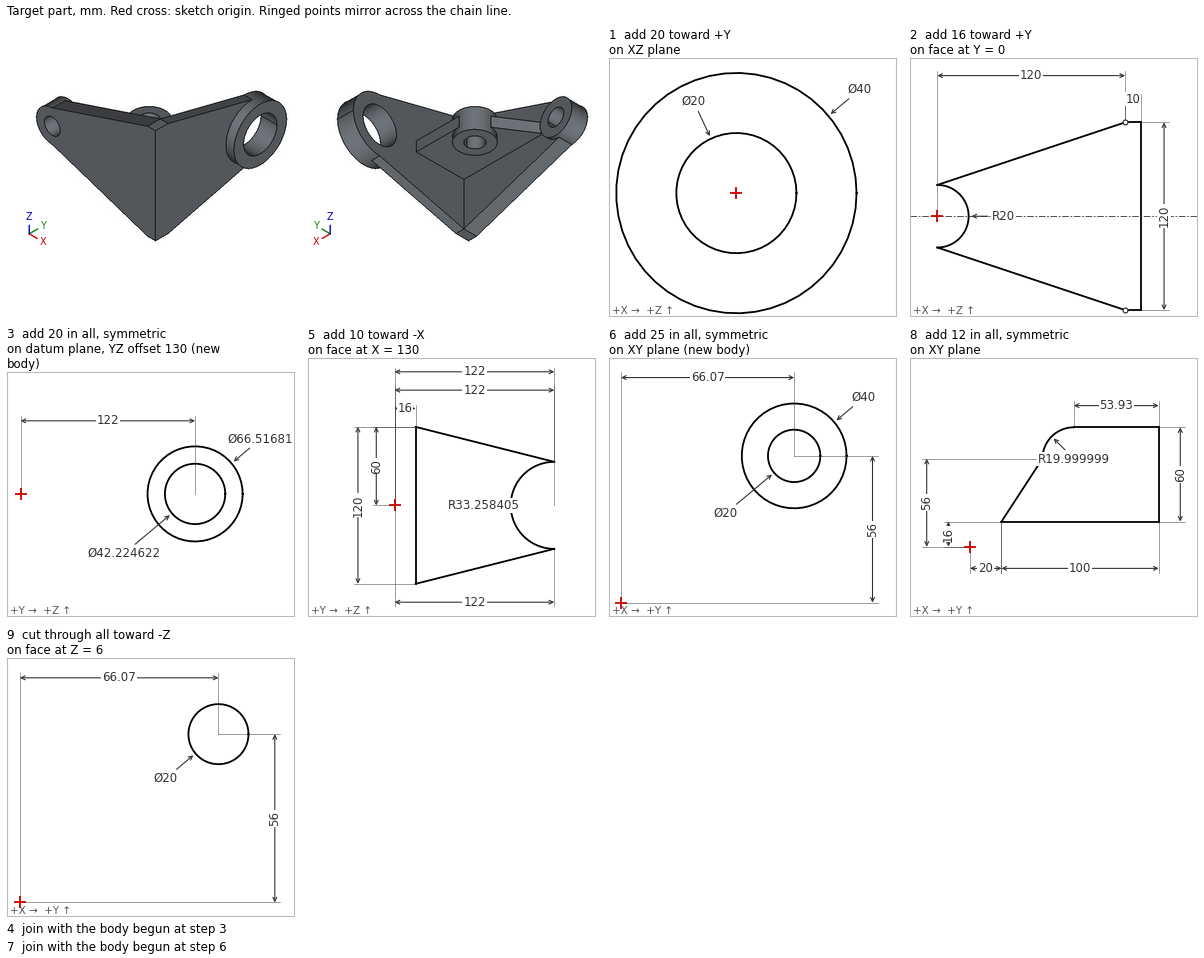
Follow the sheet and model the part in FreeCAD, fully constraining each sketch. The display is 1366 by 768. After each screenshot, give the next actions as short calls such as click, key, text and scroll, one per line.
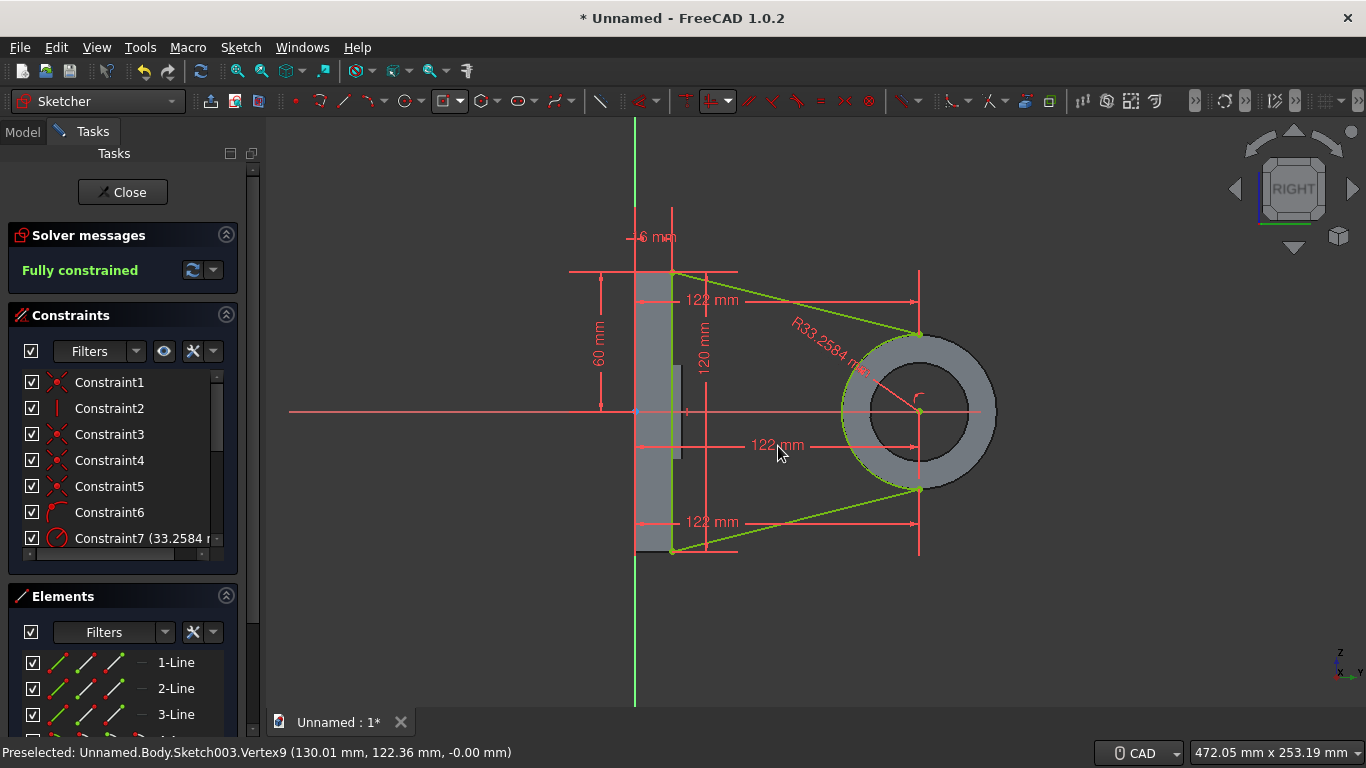
click(123, 192)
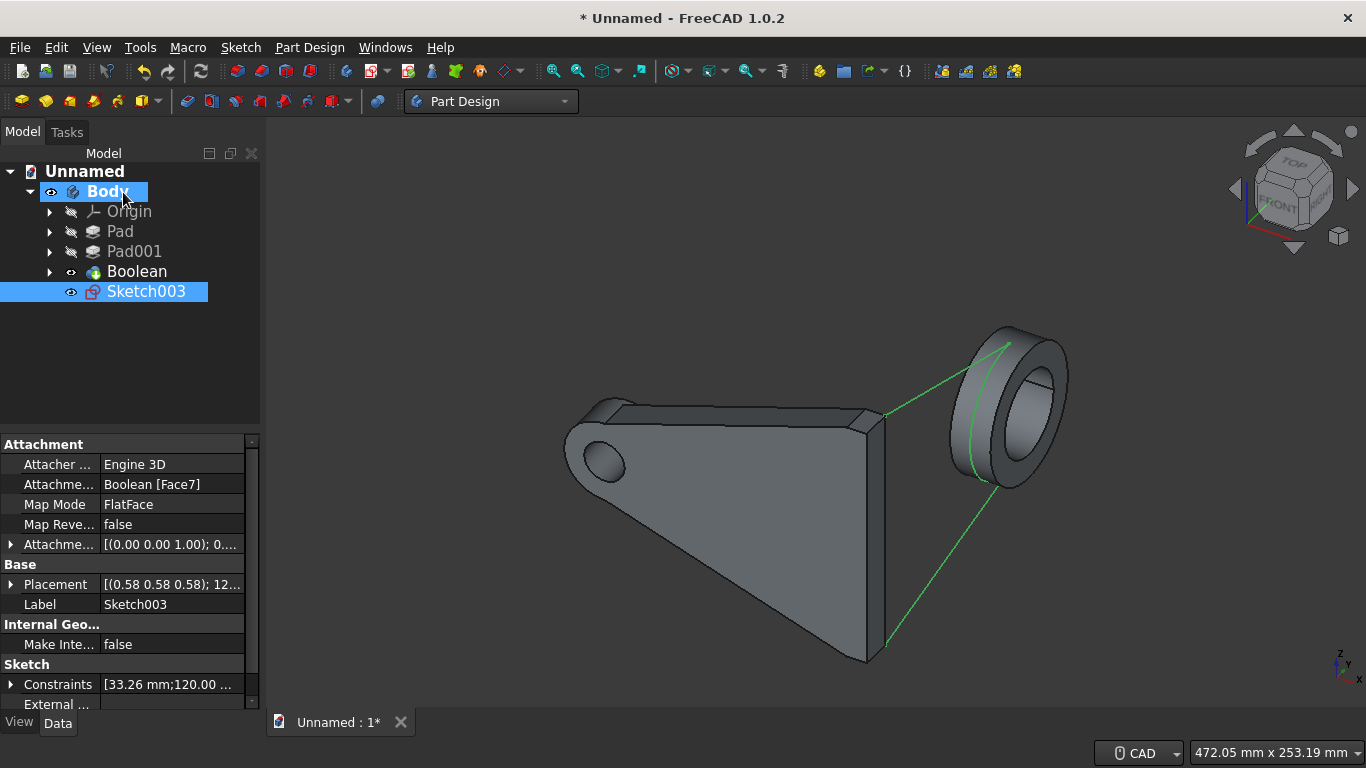
click(22, 102)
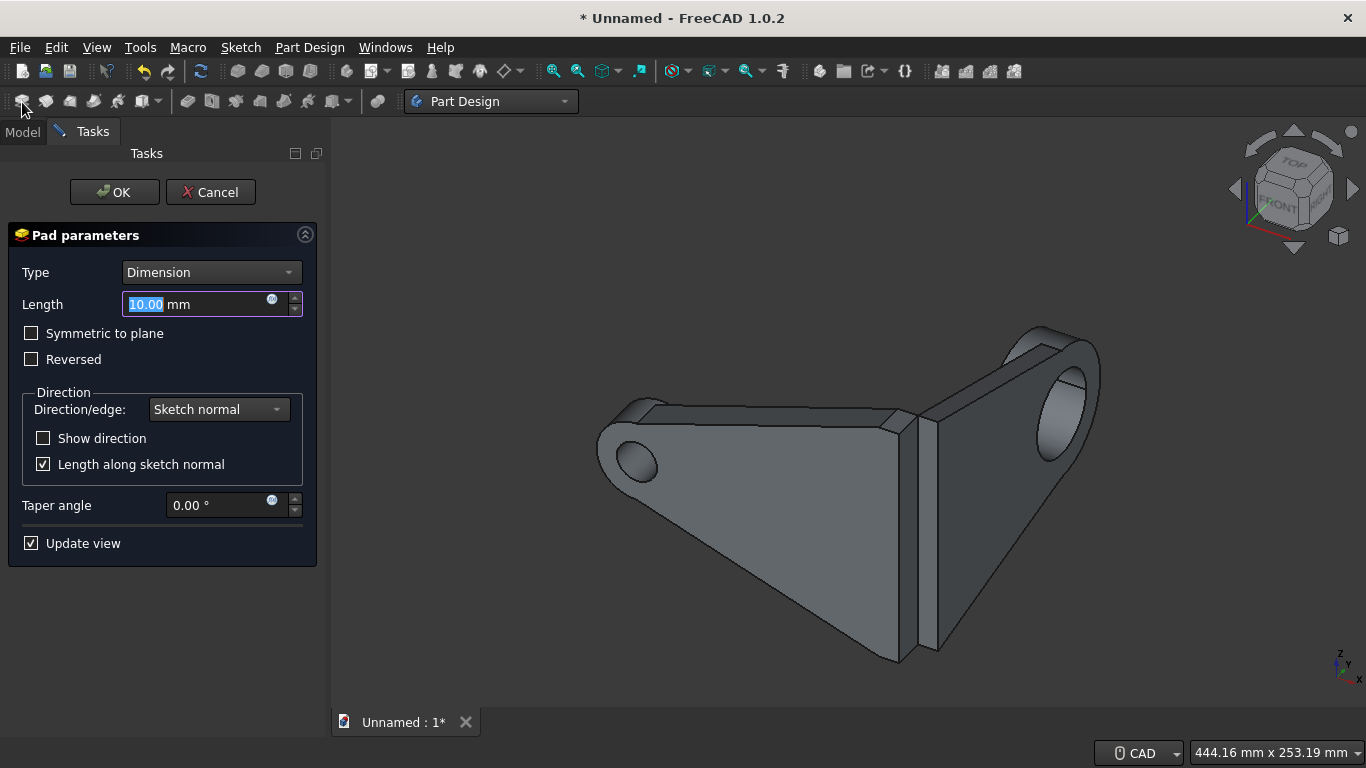
text(10)
key(Tab)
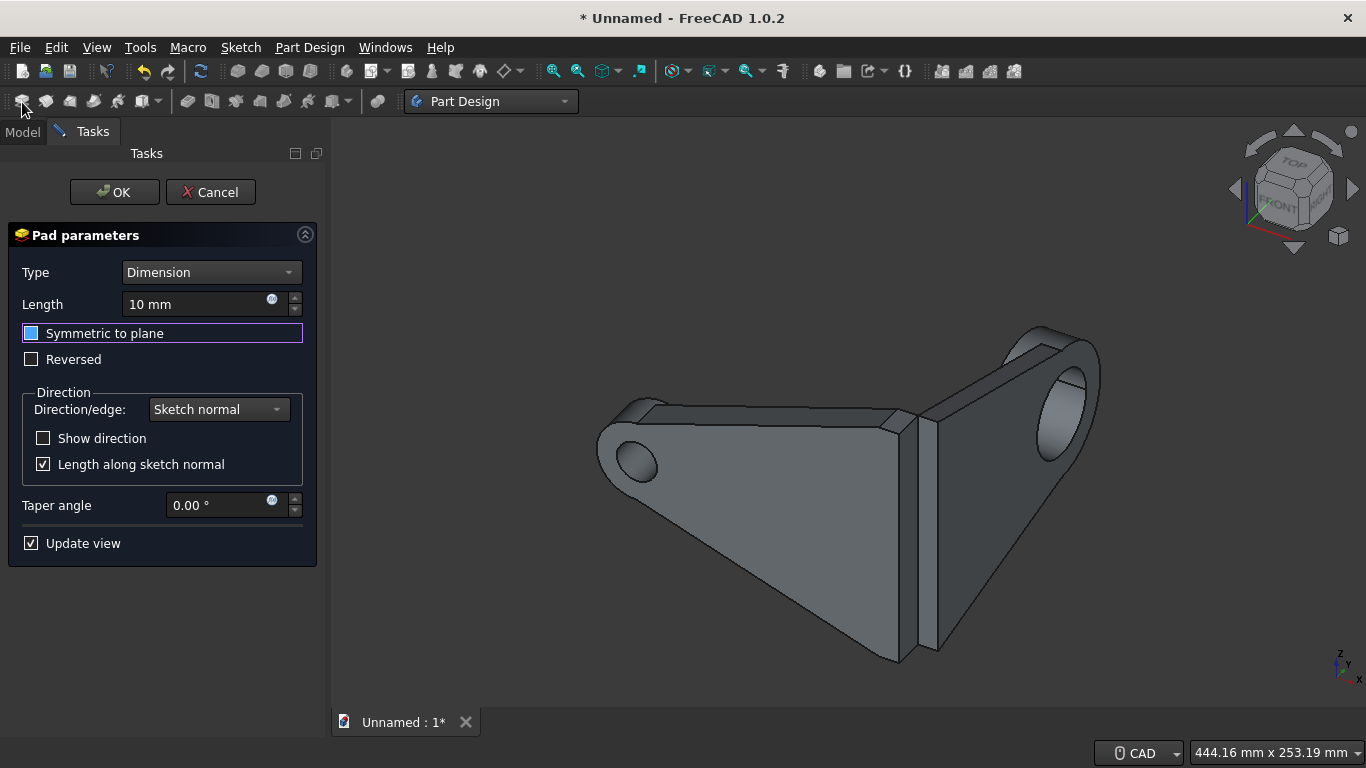
click(30, 359)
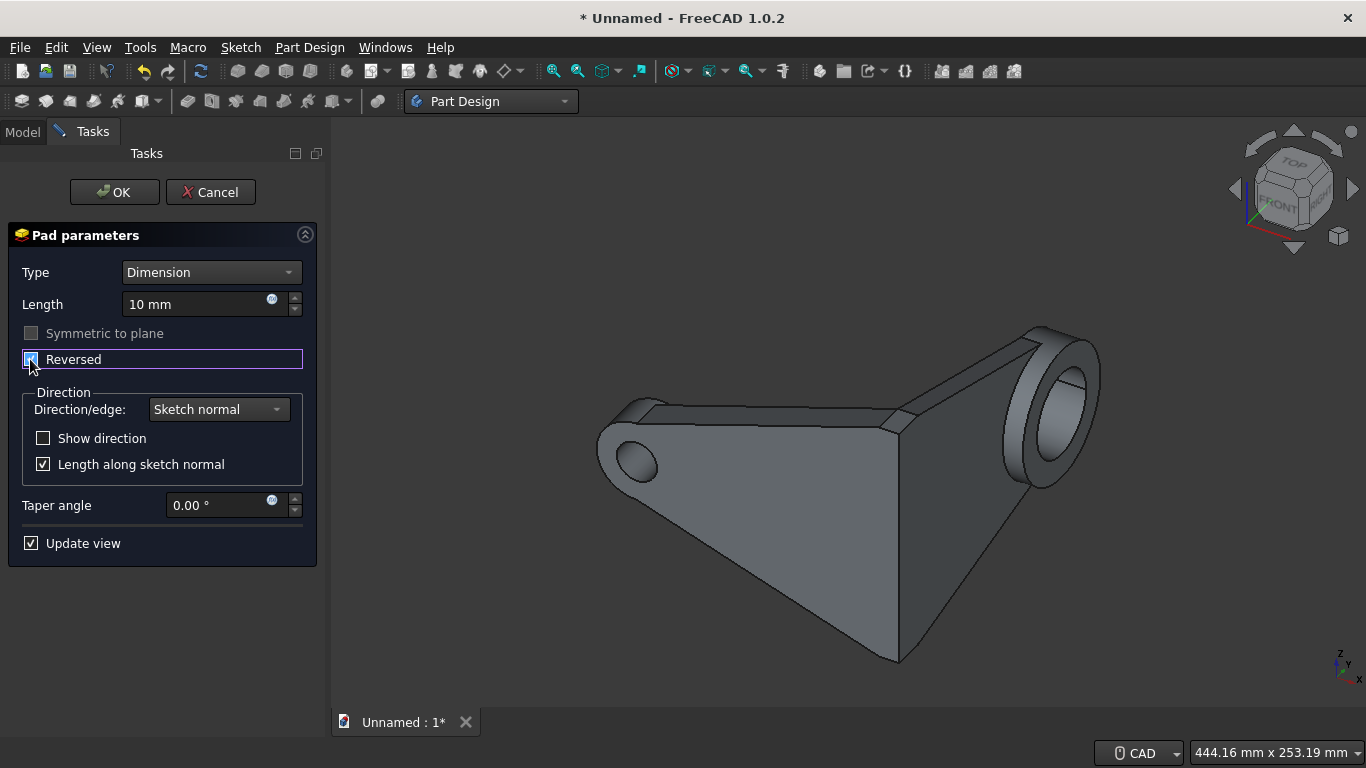
click(115, 192)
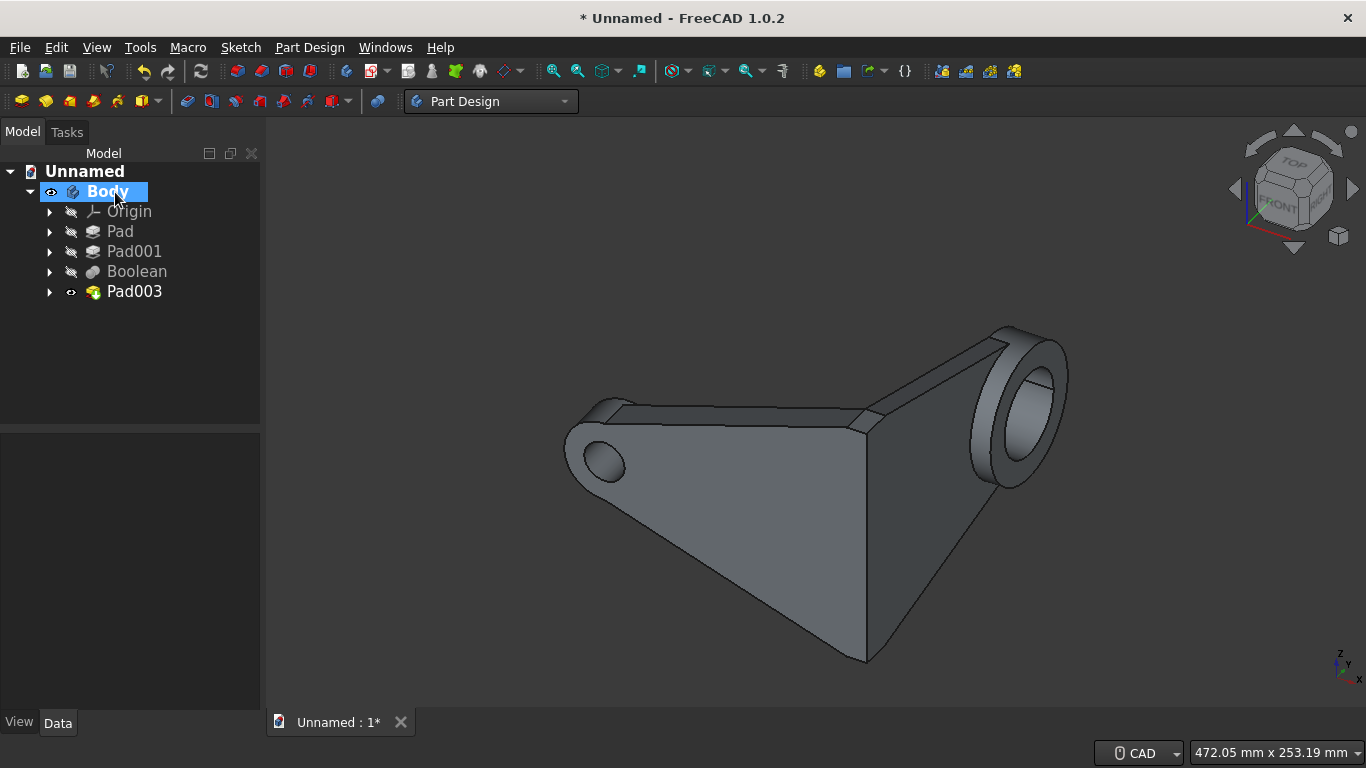
click(348, 72)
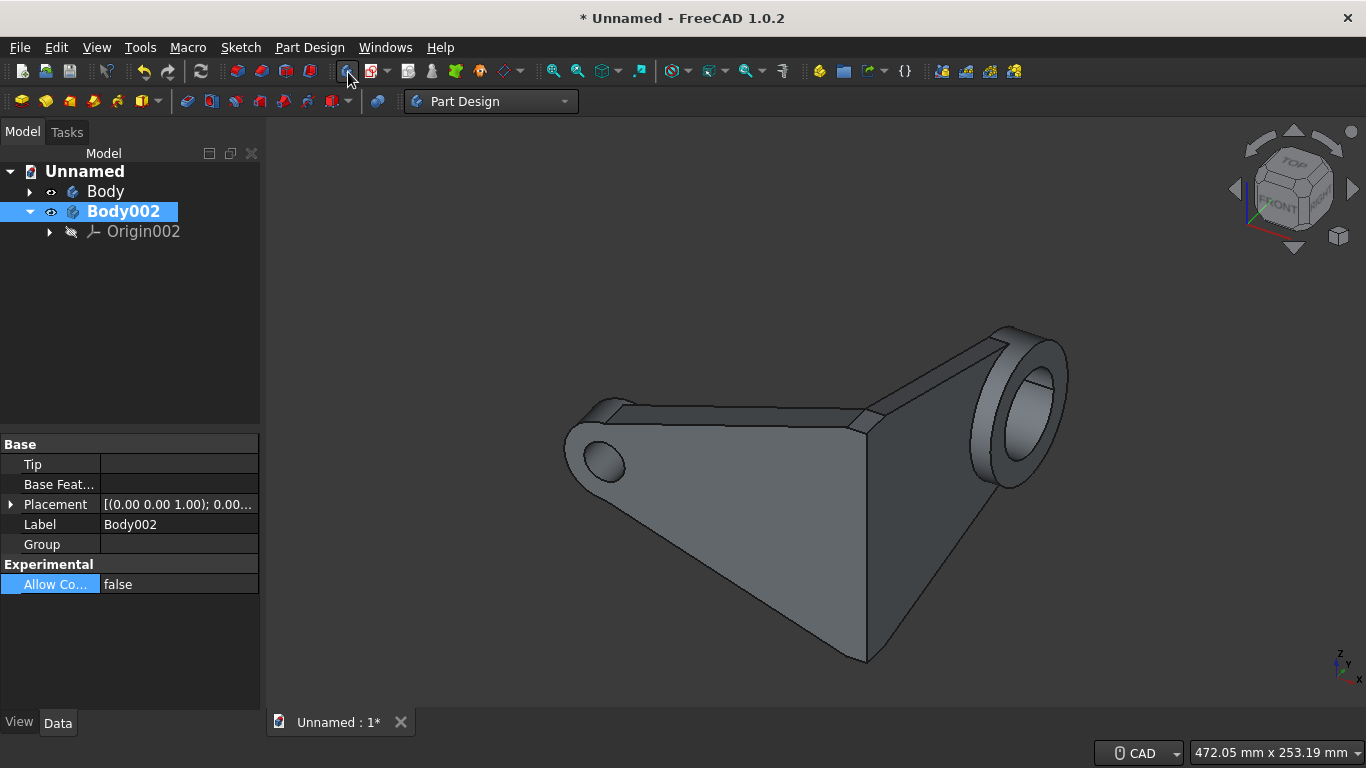
click(306, 667)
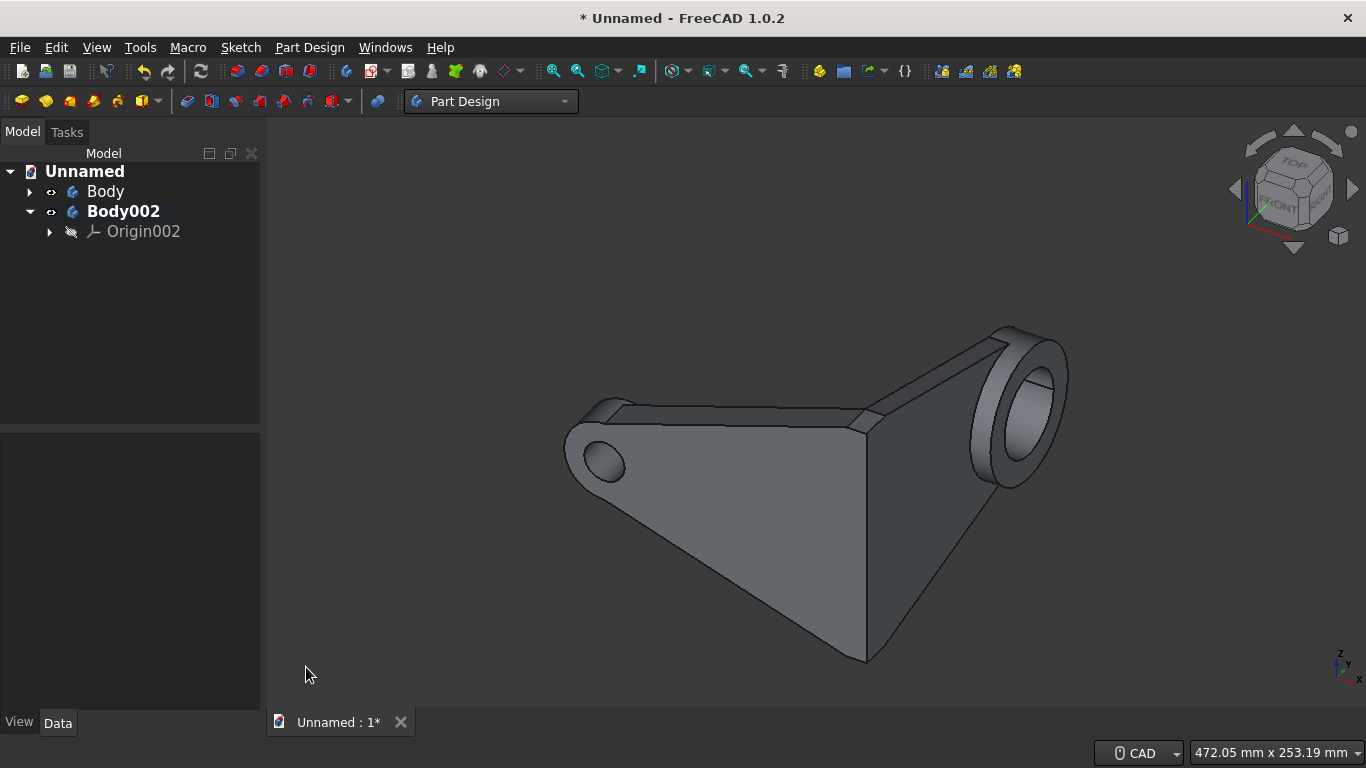
click(372, 72)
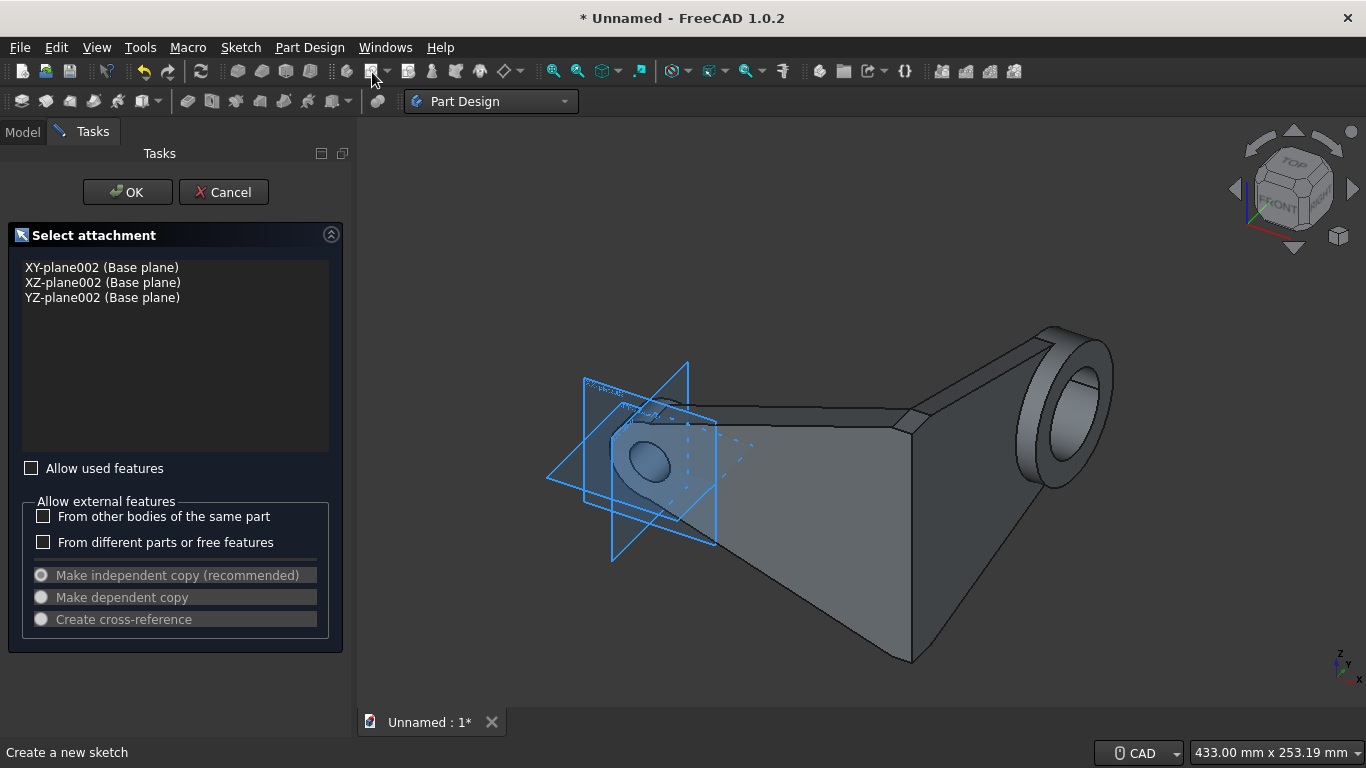
click(82, 268)